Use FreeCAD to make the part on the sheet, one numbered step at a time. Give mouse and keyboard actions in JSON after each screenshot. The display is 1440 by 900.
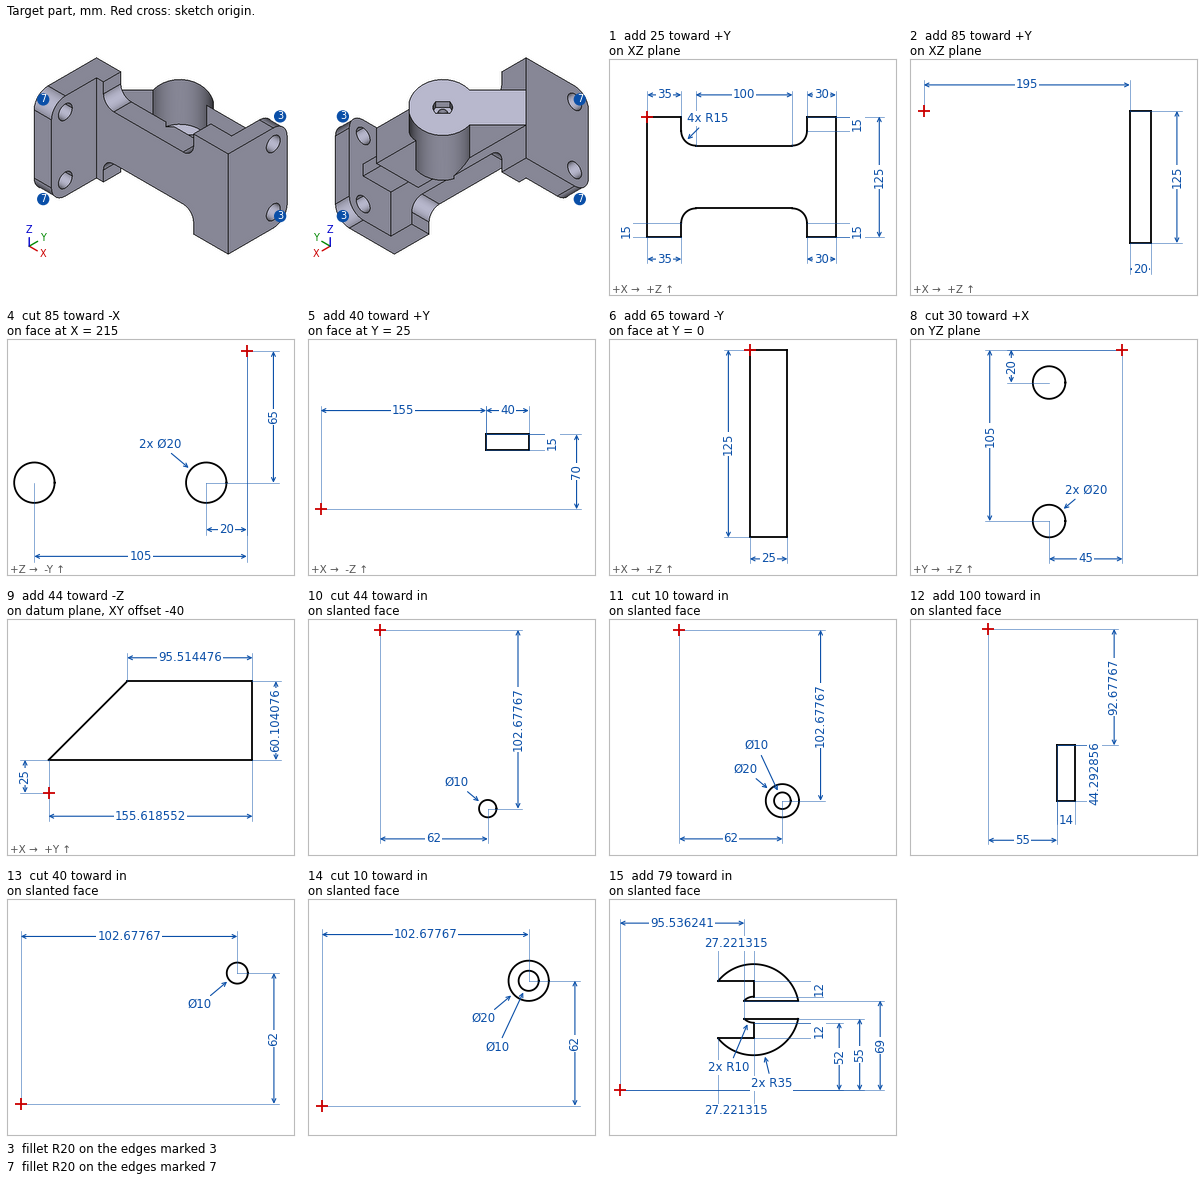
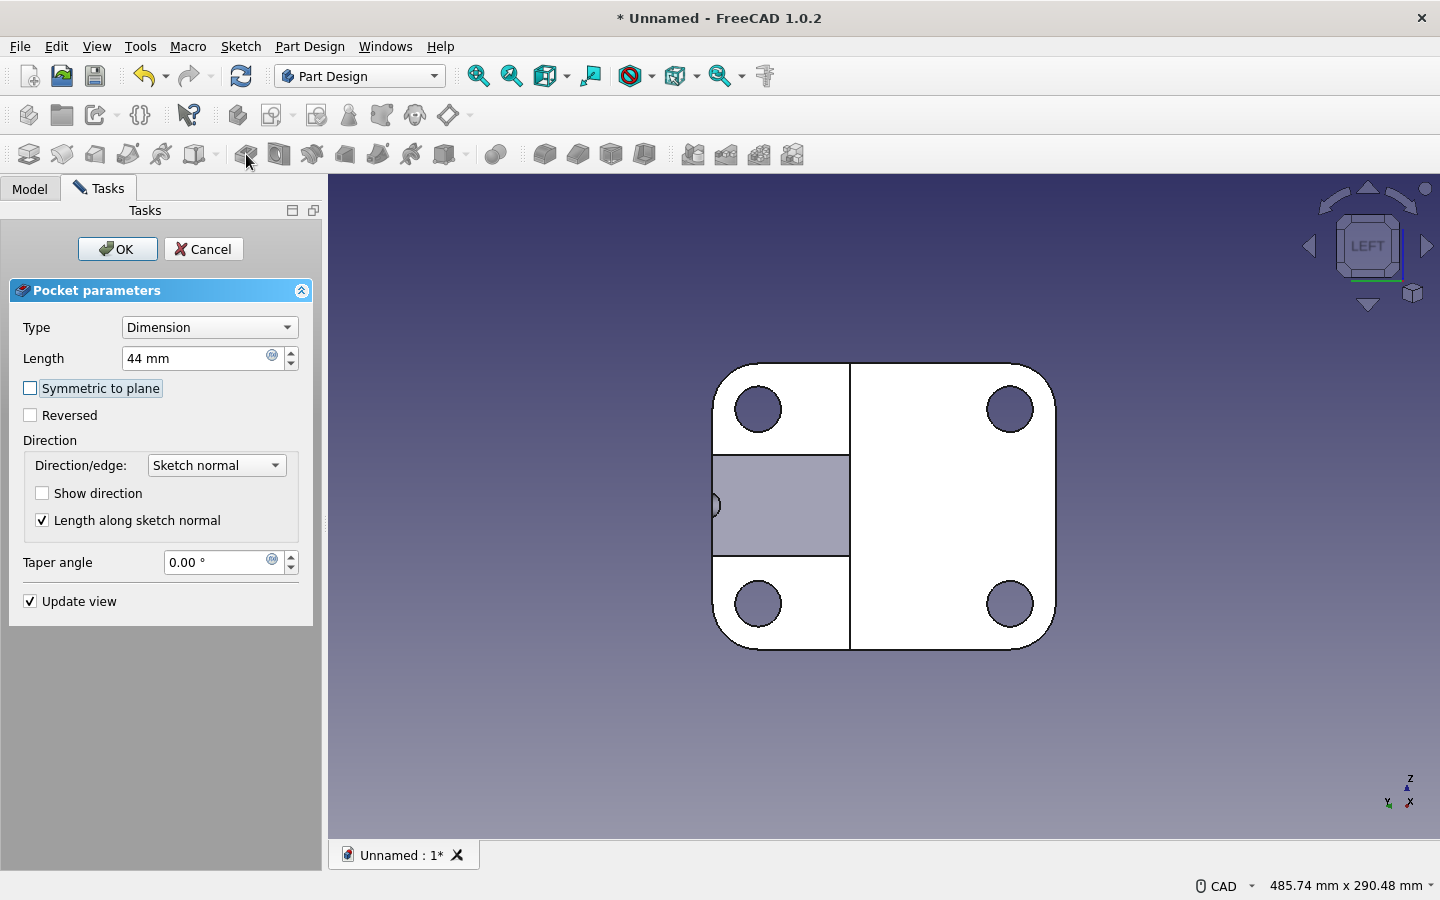
{"action": "left_click", "coordinate": [118, 249]}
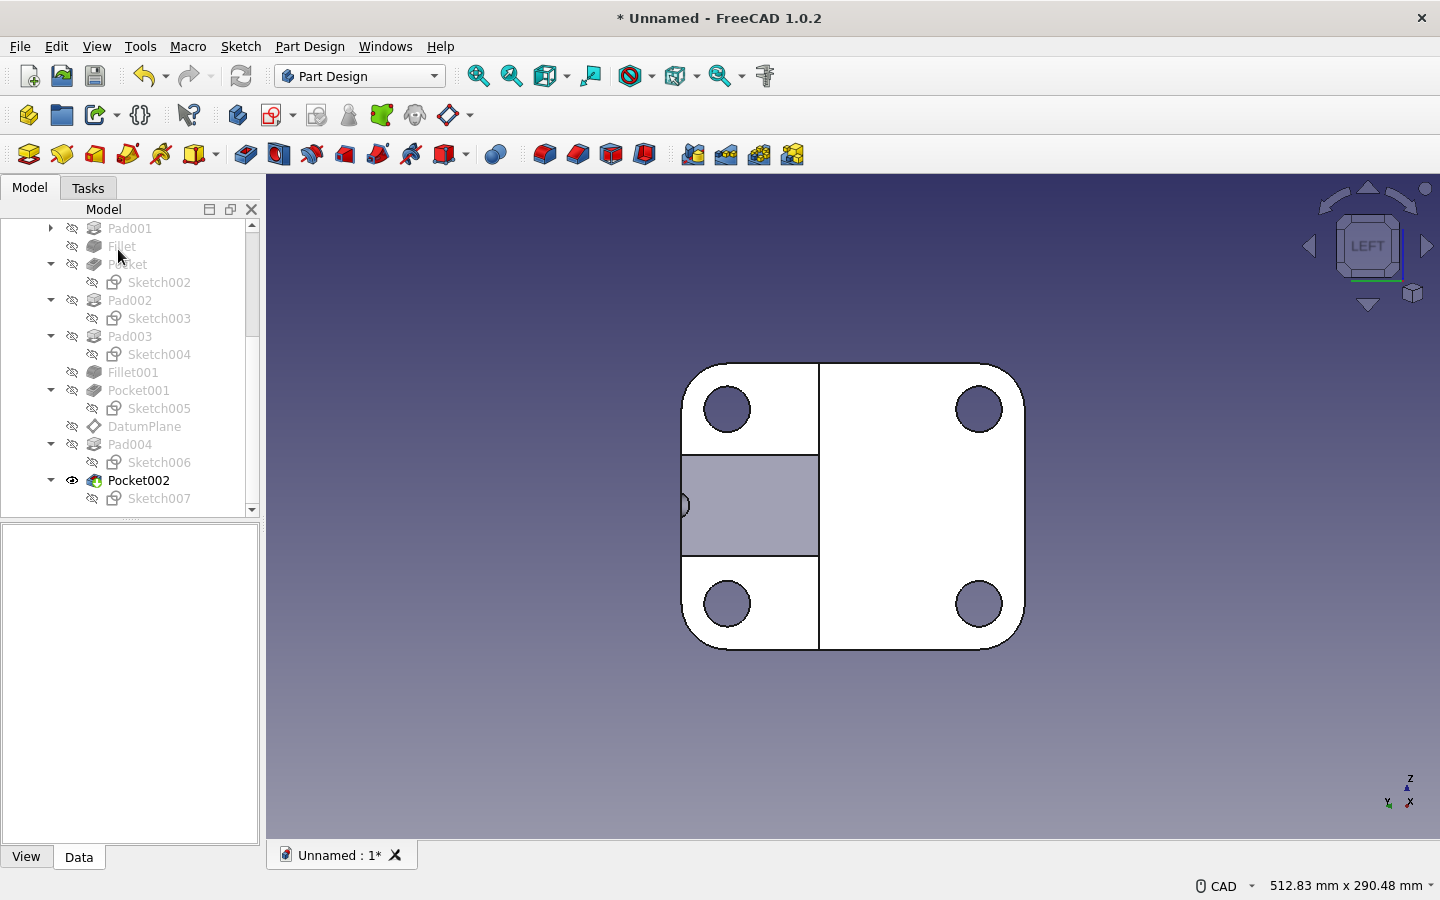
{"action": "left_click", "coordinate": [479, 76]}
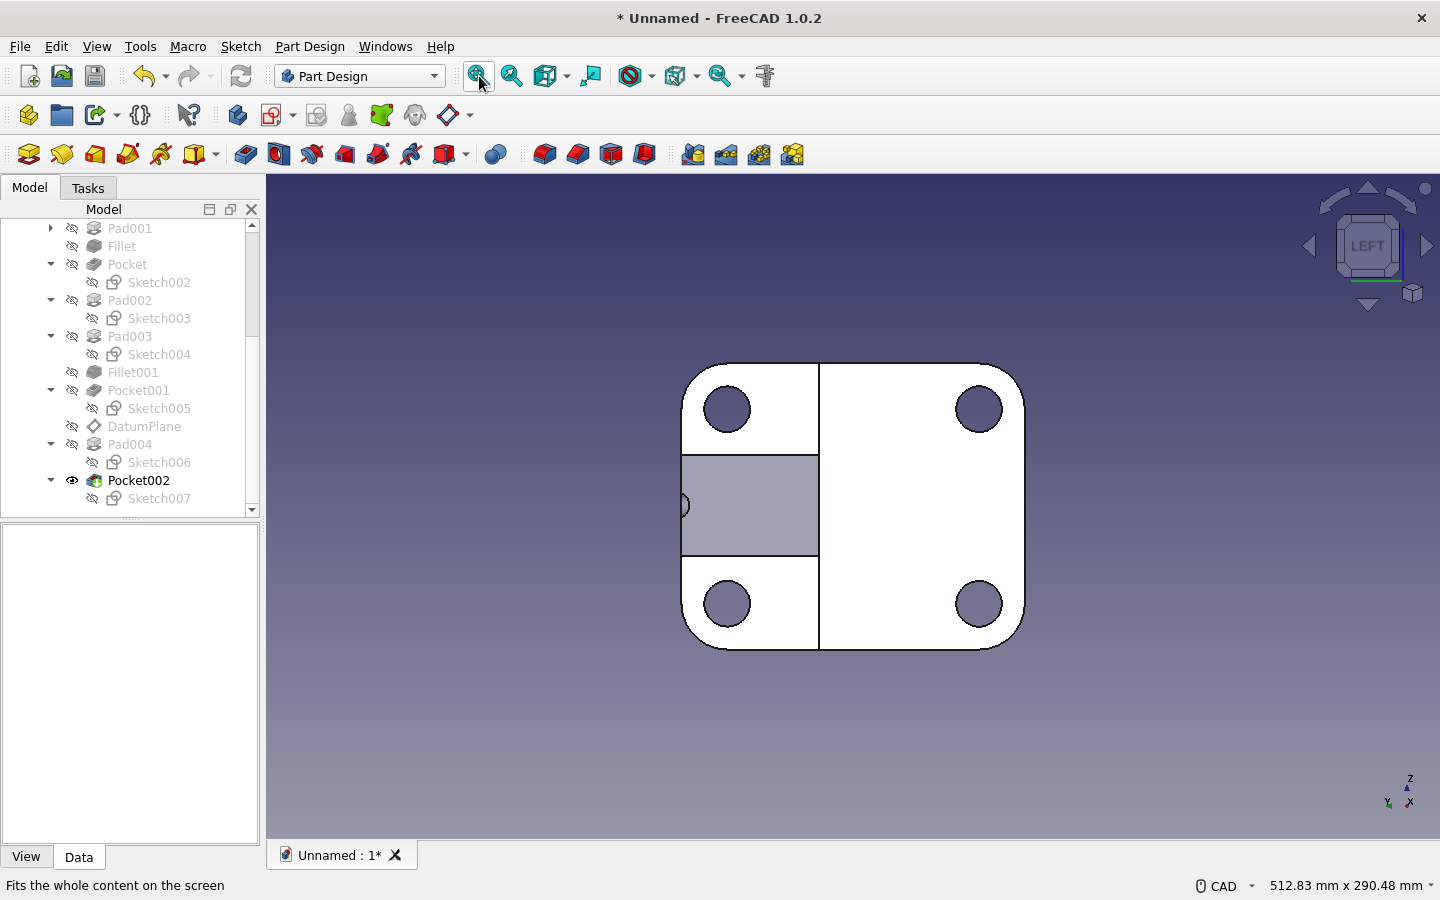
{"action": "left_click", "coordinate": [730, 504]}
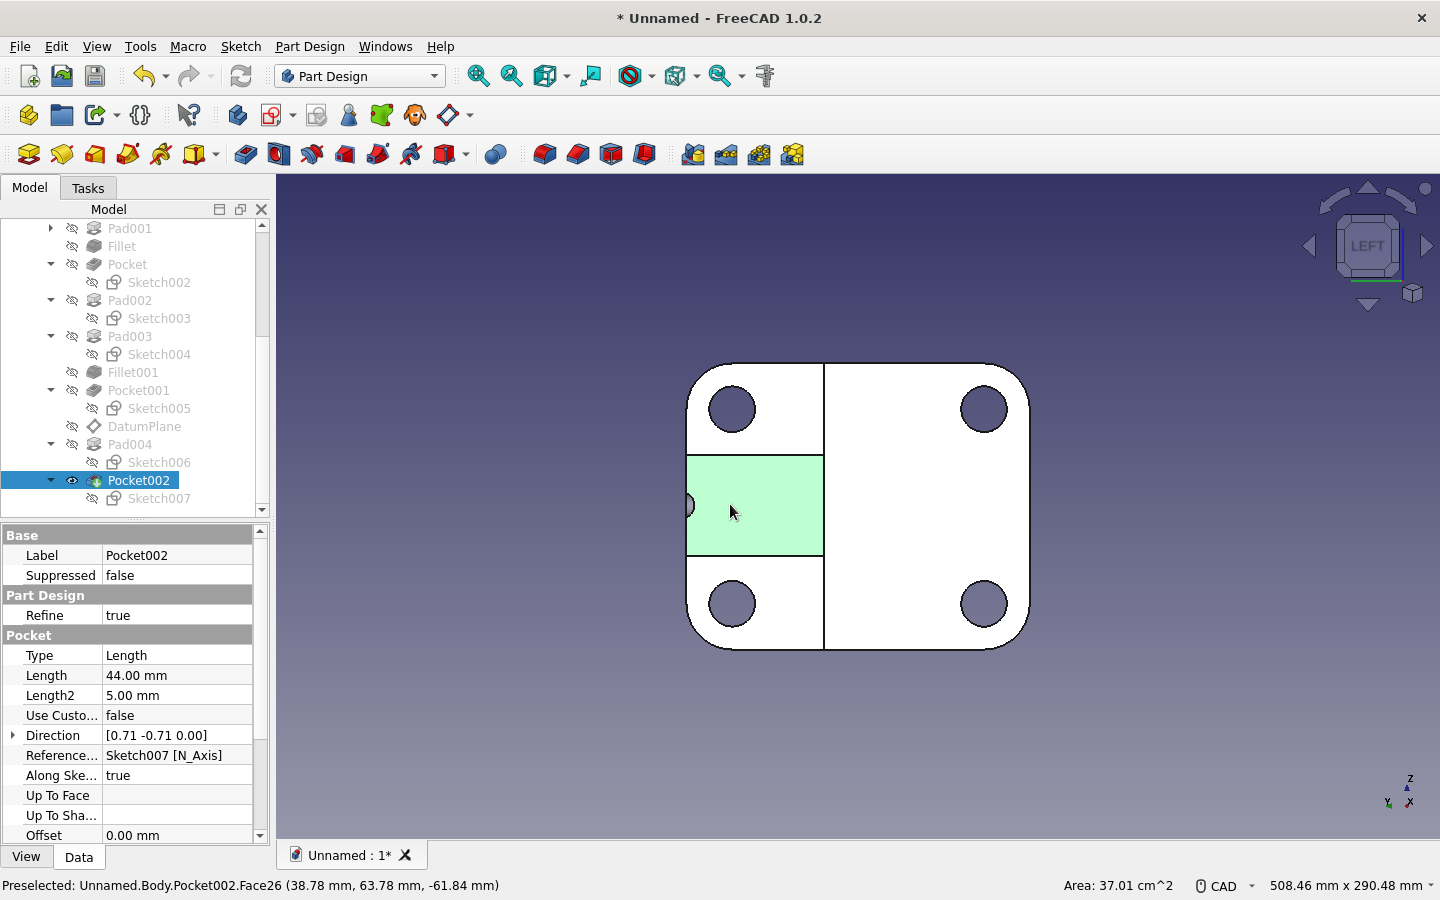
{"action": "left_click", "coordinate": [270, 116]}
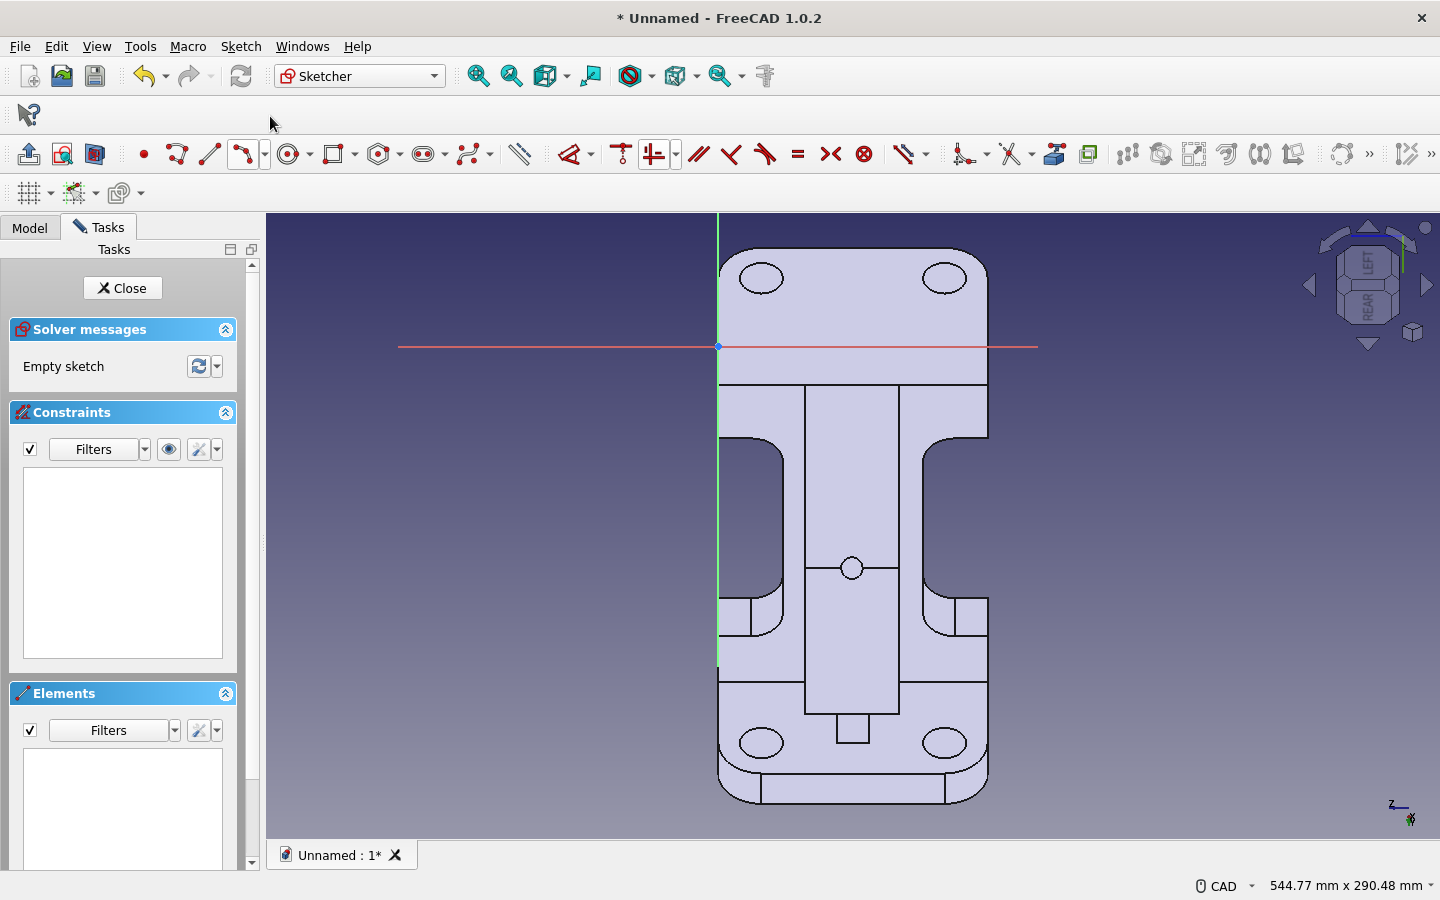
{"action": "left_click", "coordinate": [95, 154]}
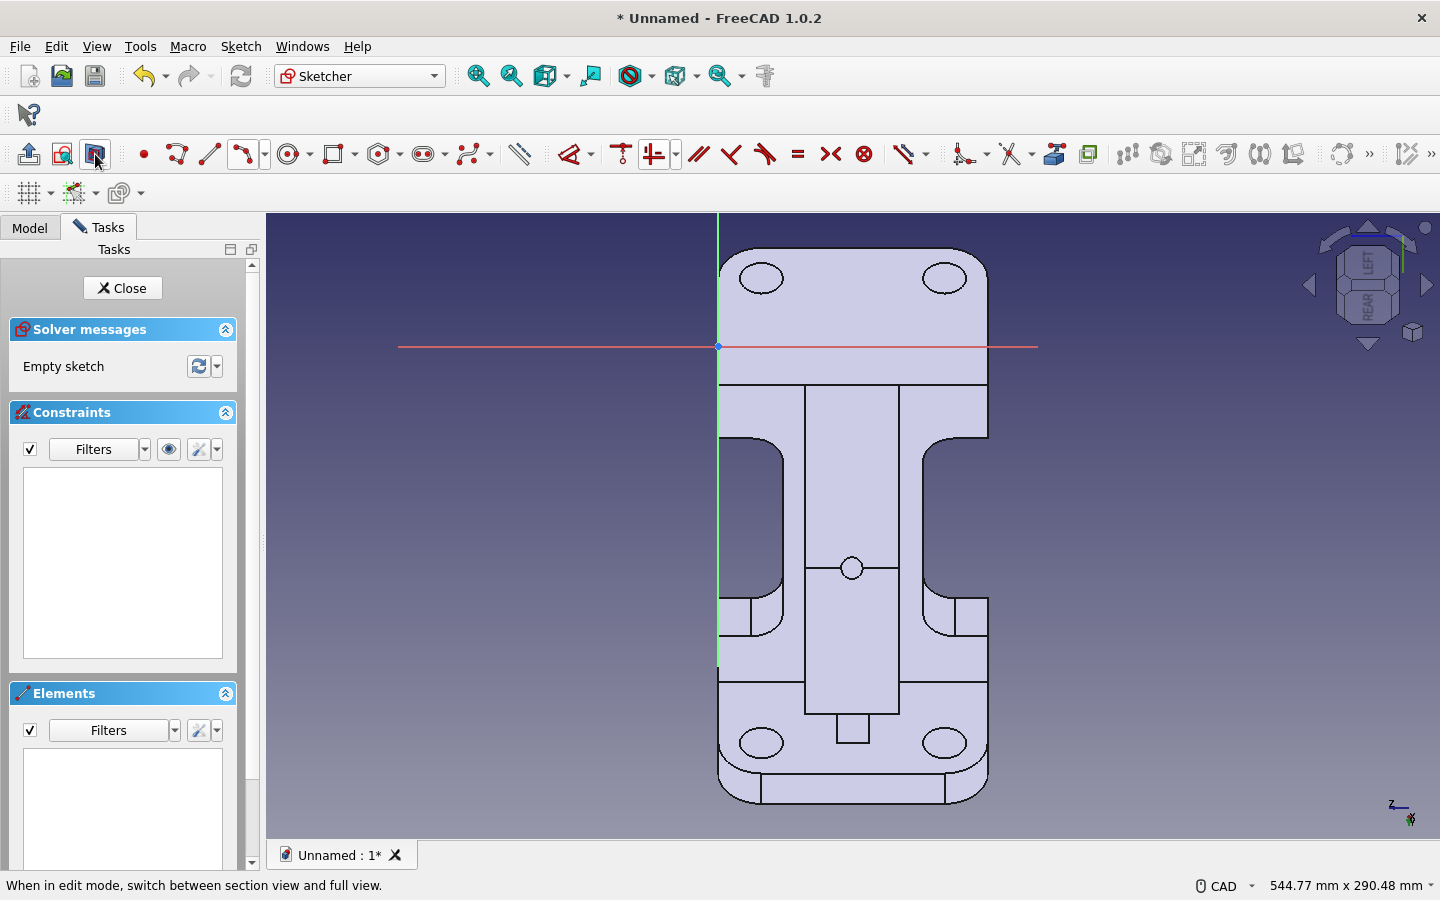
{"action": "scroll", "coordinate": [860, 573], "scroll_direction": "up", "scroll_amount": 11}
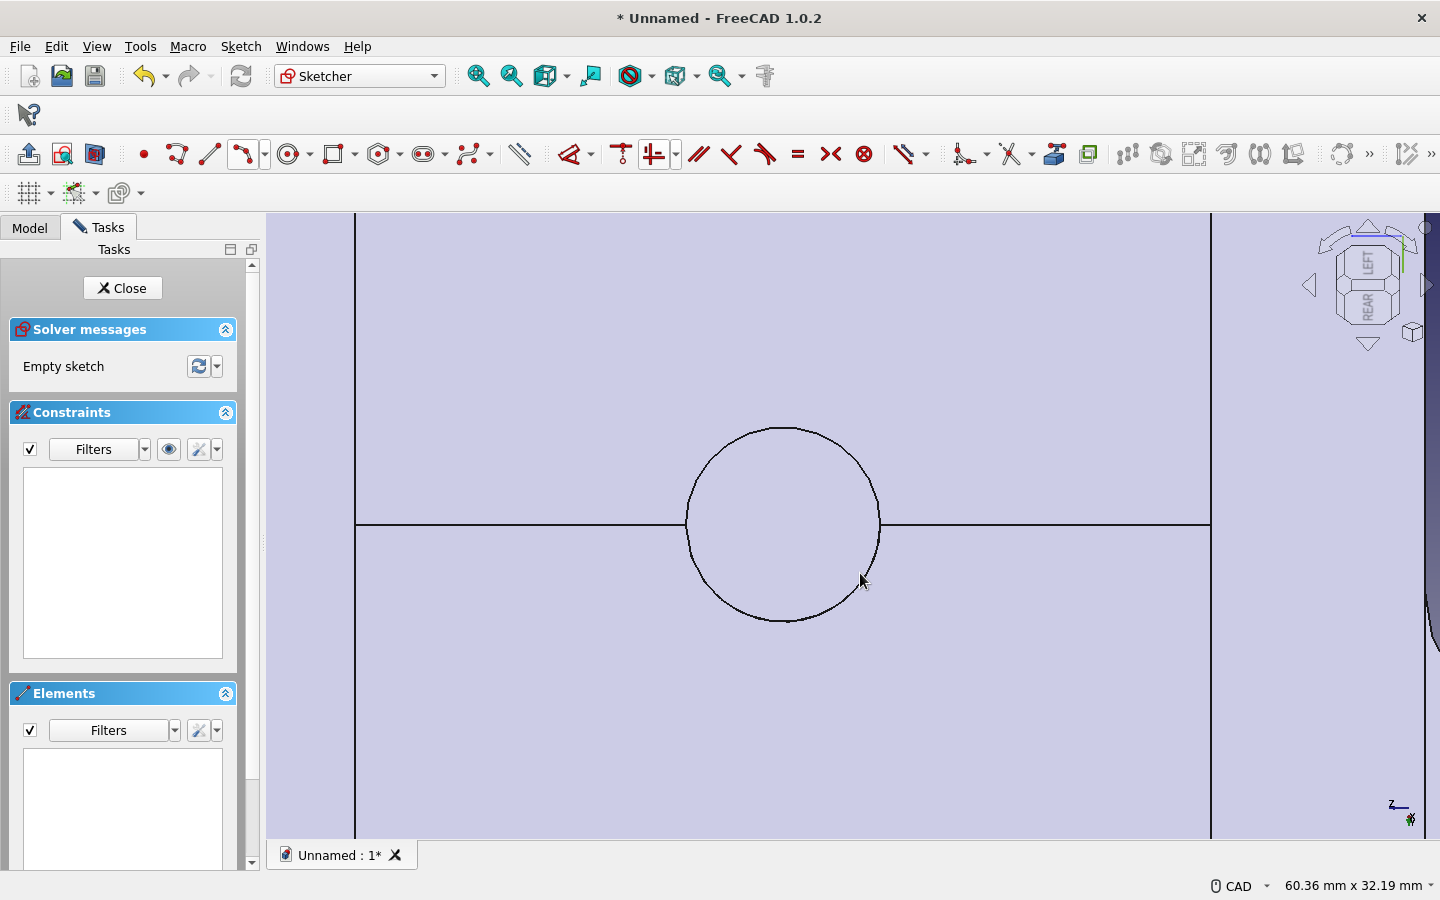
{"action": "left_click", "coordinate": [288, 154]}